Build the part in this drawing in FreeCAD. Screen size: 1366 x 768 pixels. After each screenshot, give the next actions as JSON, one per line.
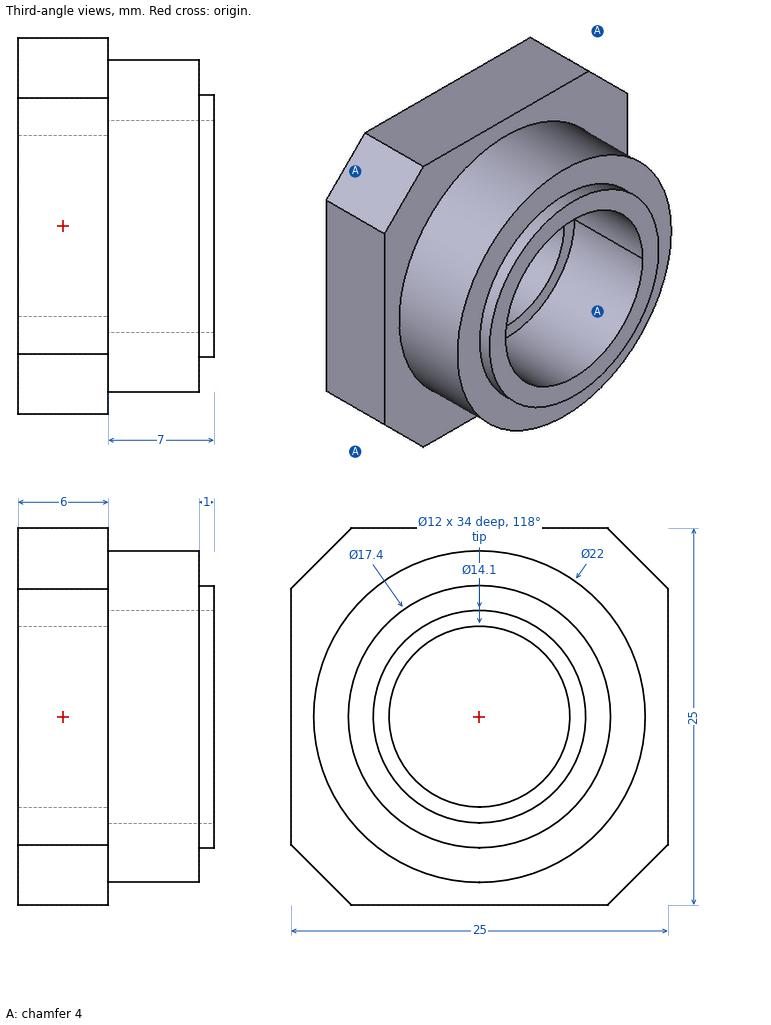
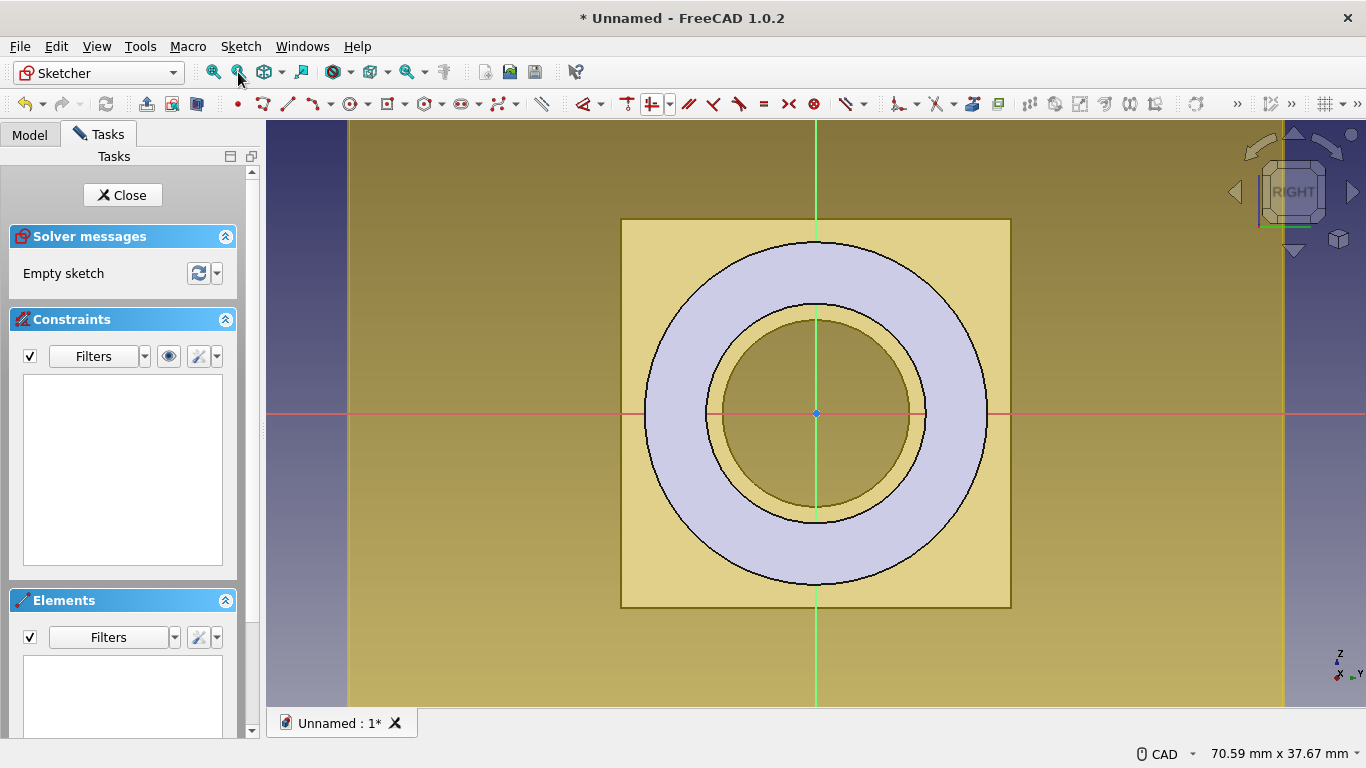
{"action": "left_click", "coordinate": [197, 104]}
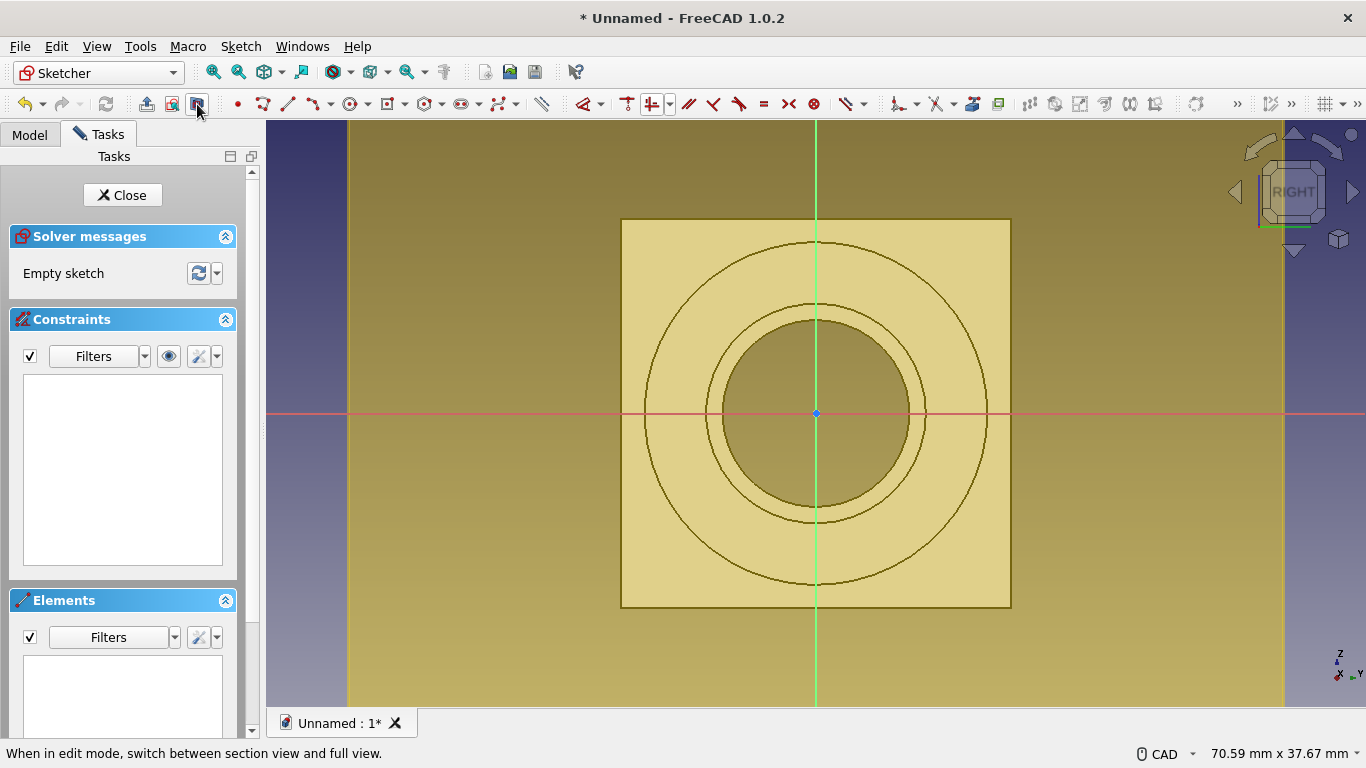
{"action": "left_click", "coordinate": [350, 104]}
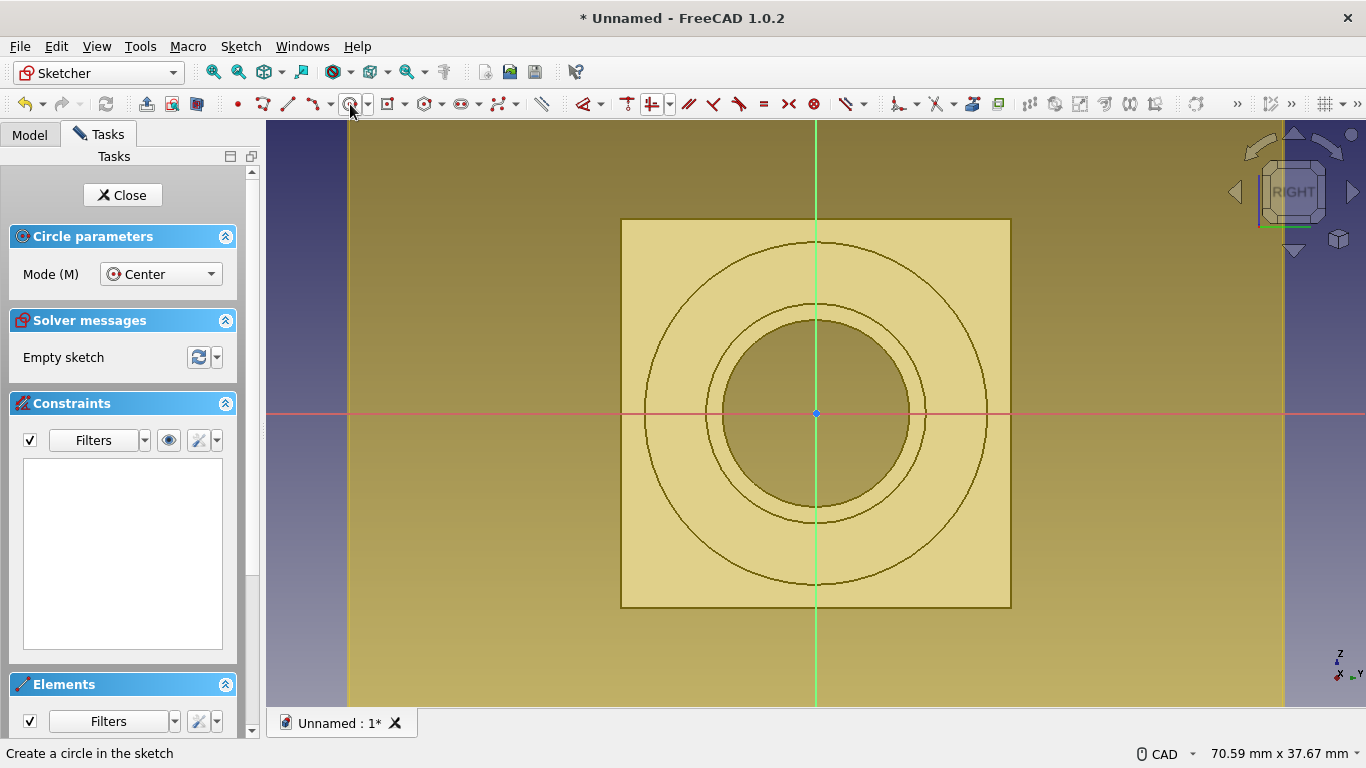
{"action": "left_click", "coordinate": [816, 414]}
{"action": "mouse_move", "coordinate": [937, 292]}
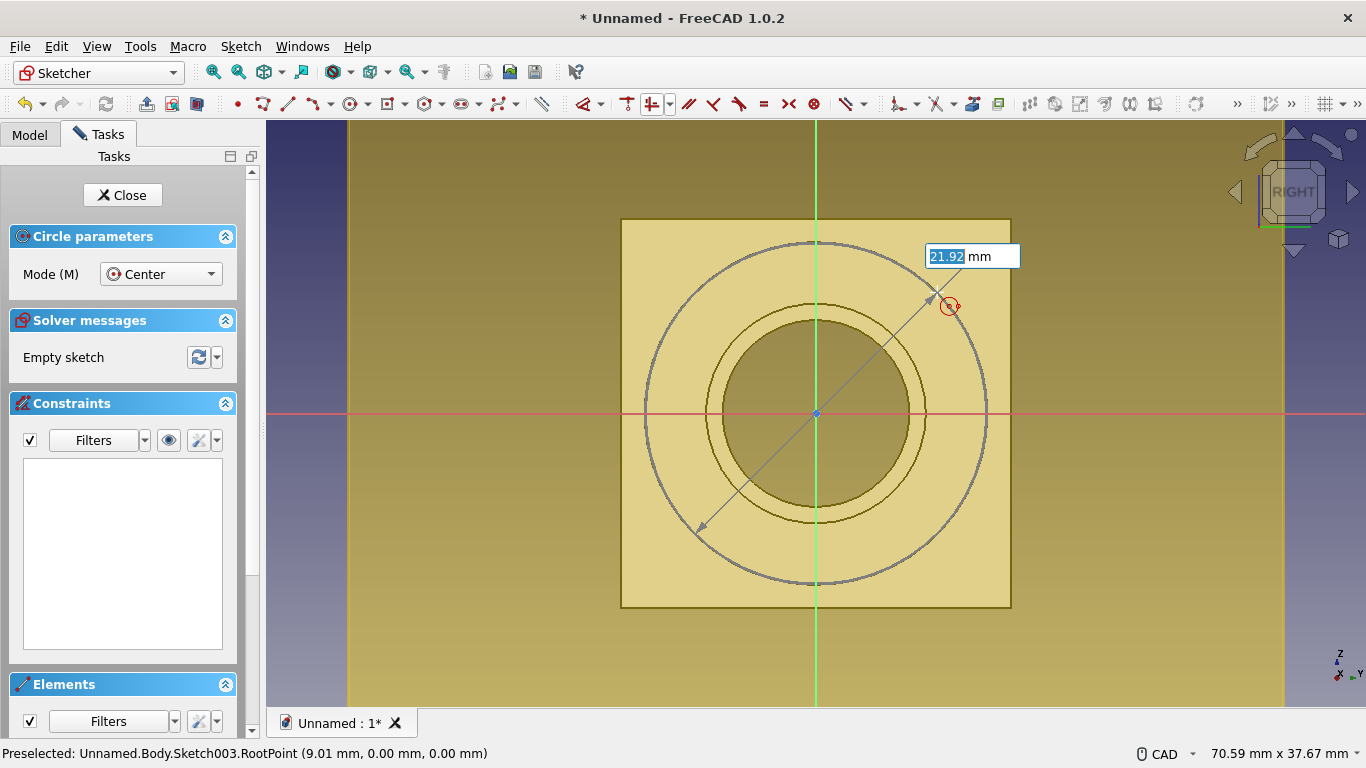
{"action": "type", "text": "22"}
{"action": "key", "text": "Return"}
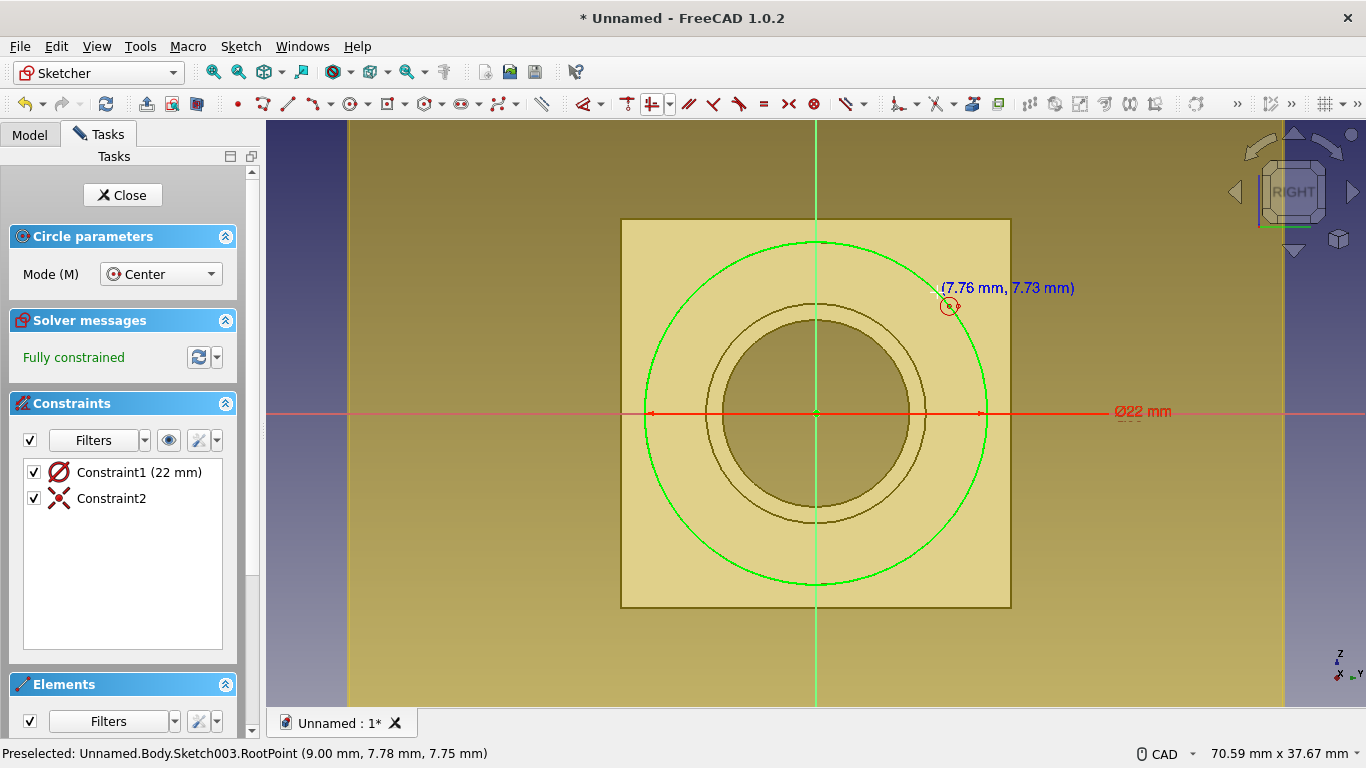
{"action": "left_click", "coordinate": [816, 414]}
{"action": "mouse_move", "coordinate": [912, 318]}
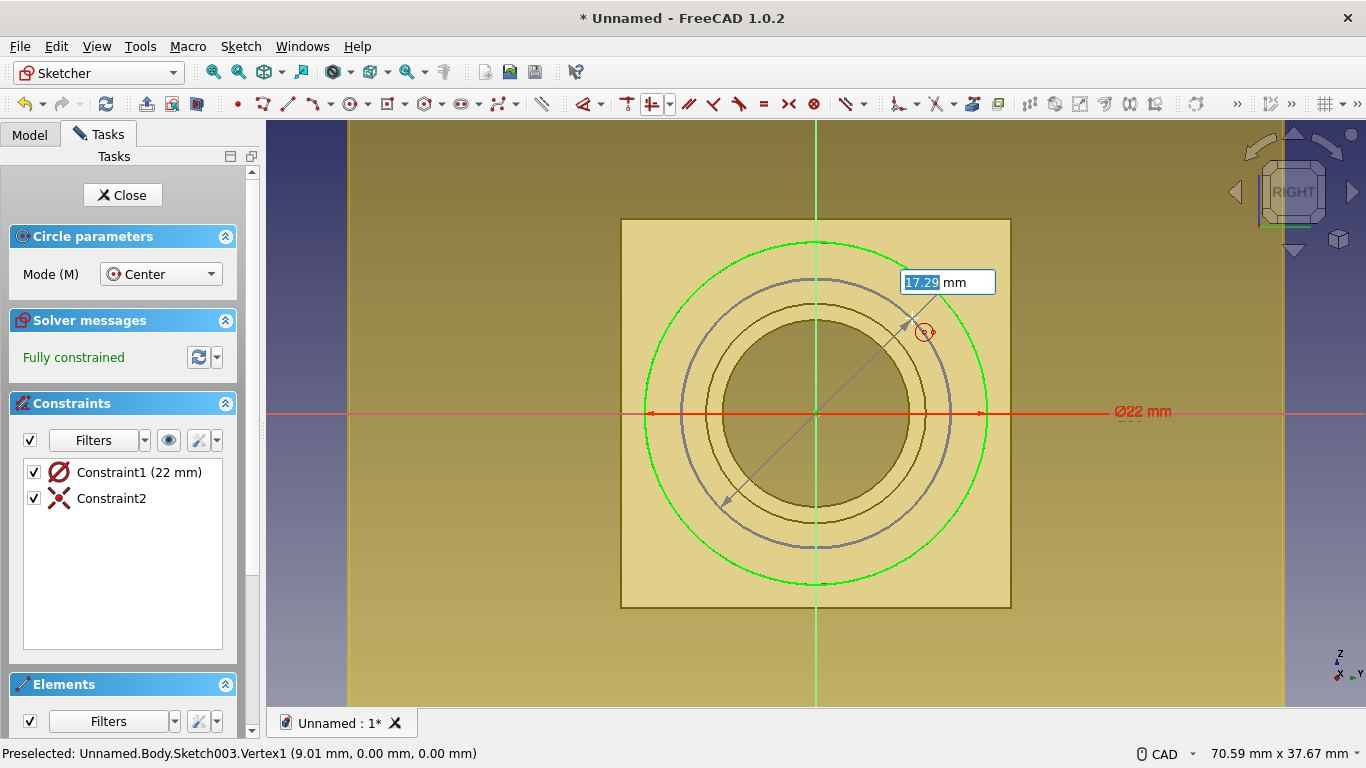
{"action": "type", "text": "17.4"}
{"action": "key", "text": "Return"}
{"action": "key", "text": "Escape"}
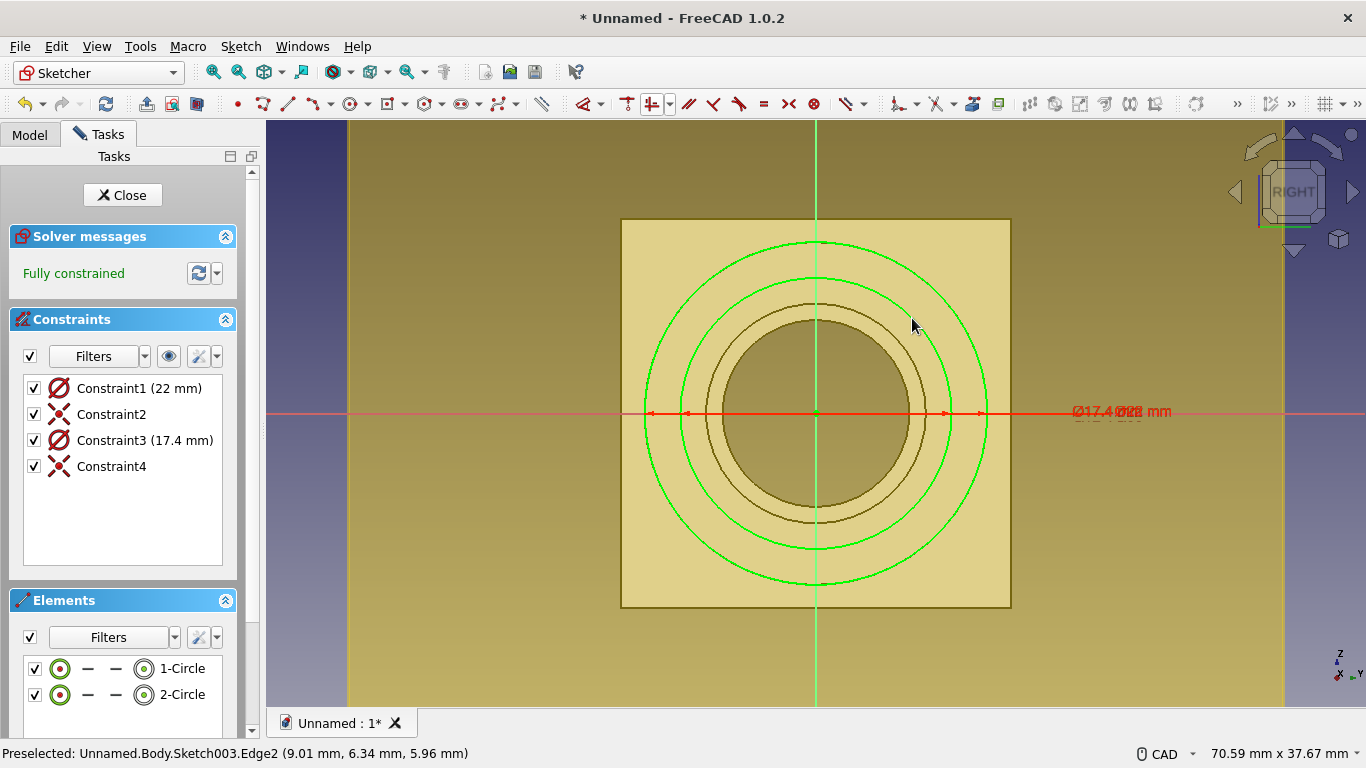
{"action": "left_click", "coordinate": [123, 195]}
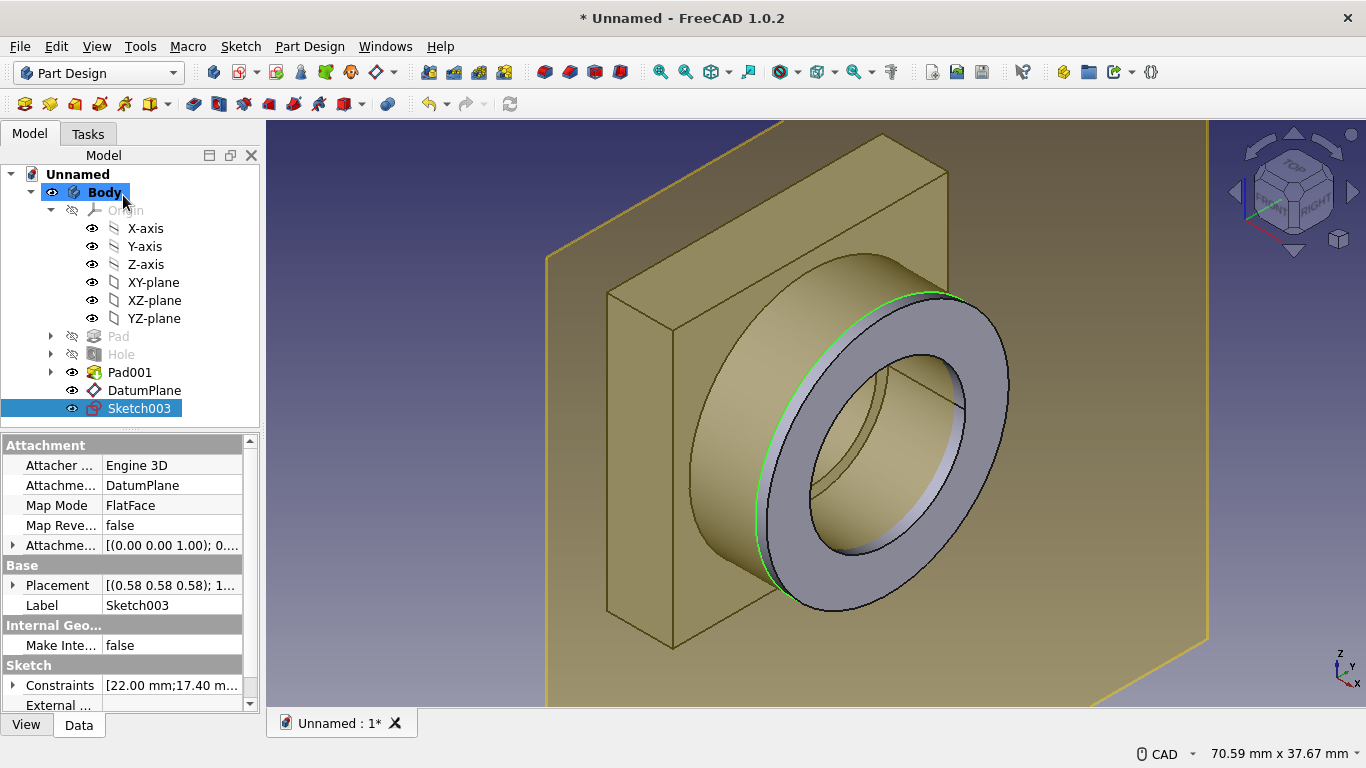
{"action": "left_click", "coordinate": [194, 104]}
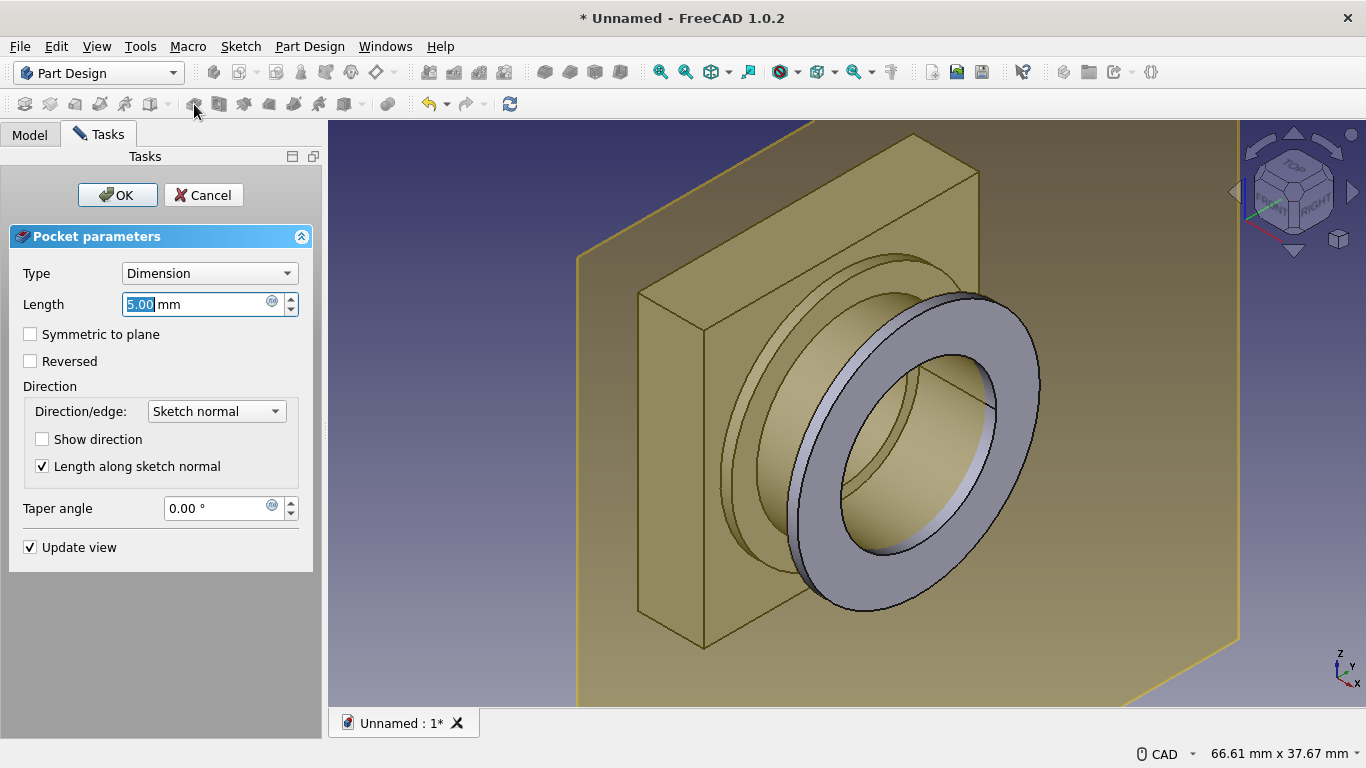
{"action": "type", "text": "1"}
{"action": "key", "text": "Tab"}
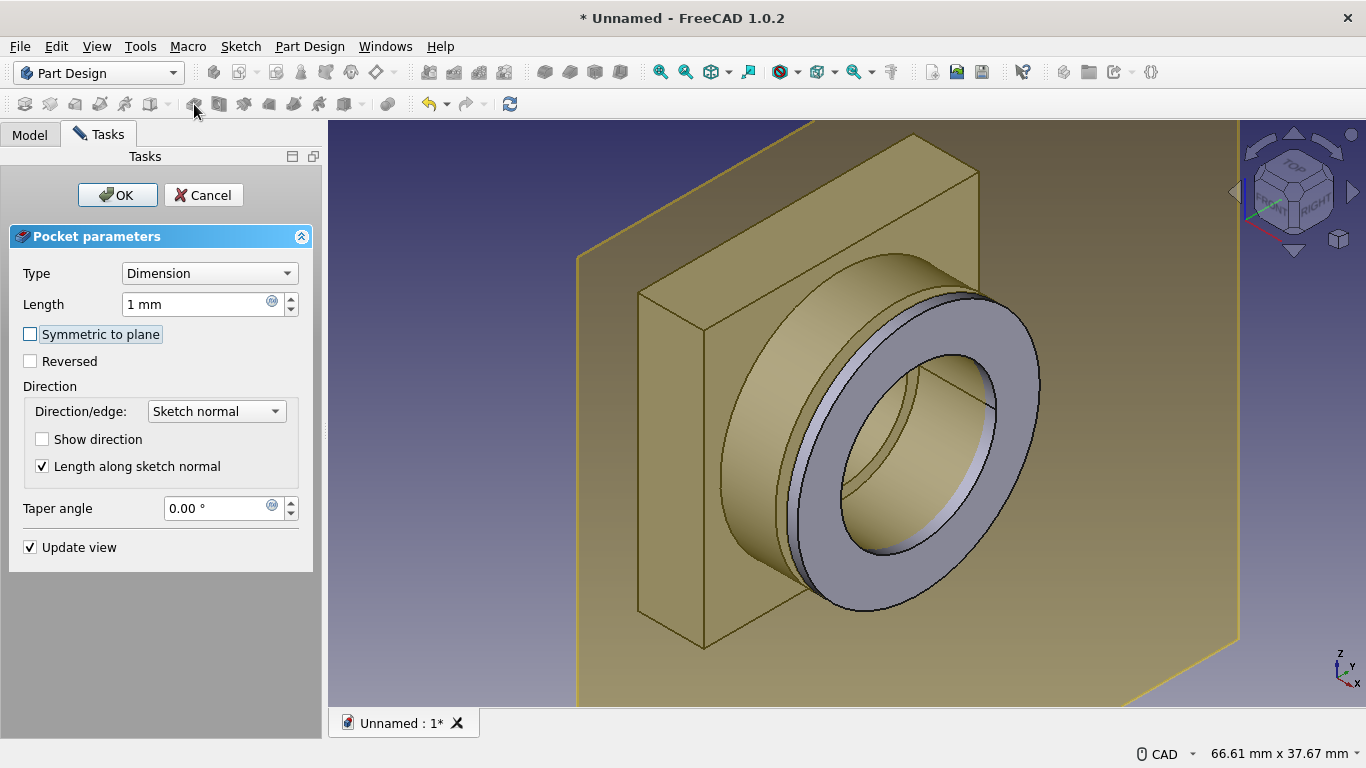
{"action": "left_click", "coordinate": [31, 361]}